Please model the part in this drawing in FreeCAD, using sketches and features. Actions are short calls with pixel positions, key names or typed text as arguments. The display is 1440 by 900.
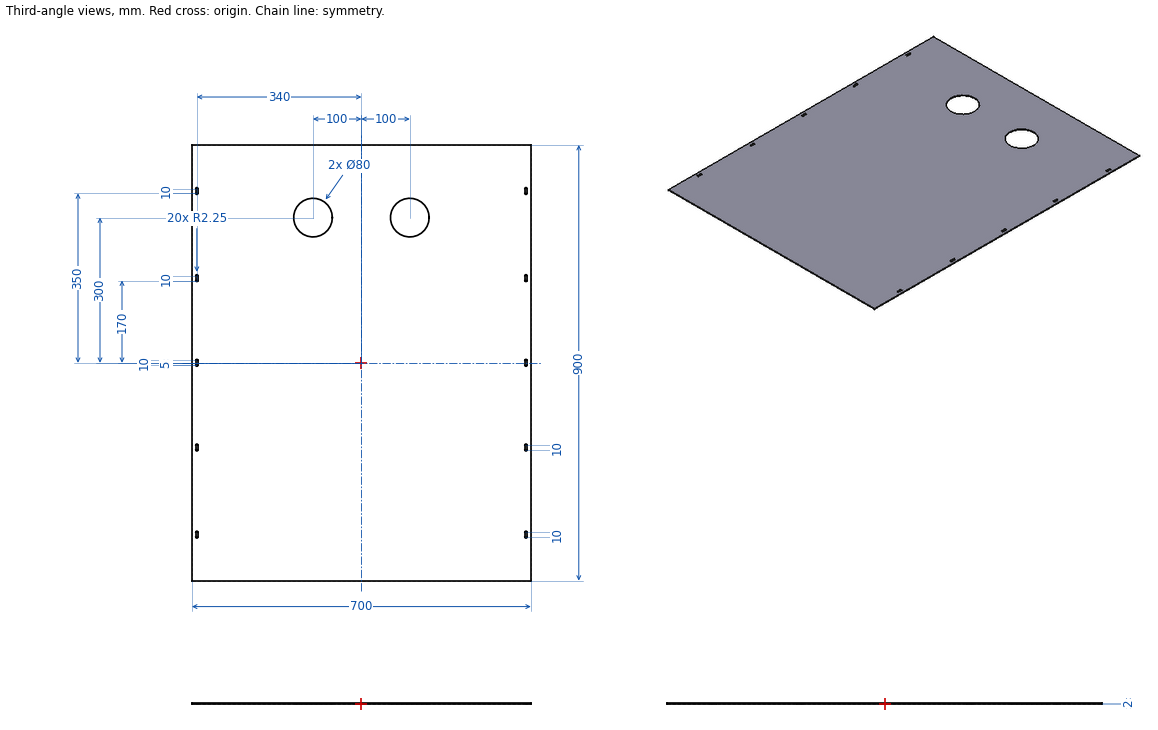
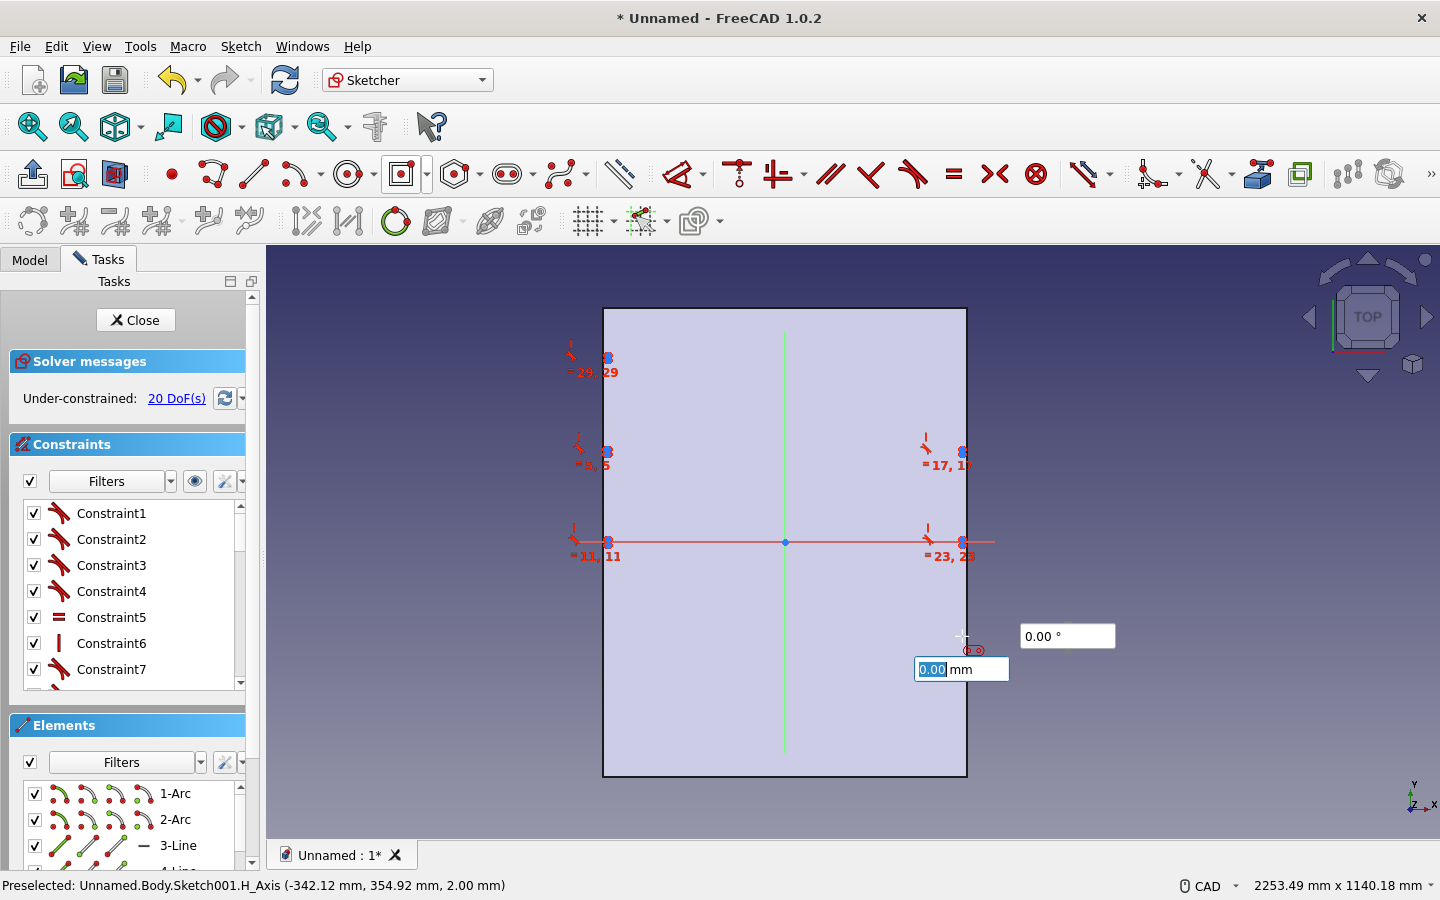
scroll(962, 631, up, 6)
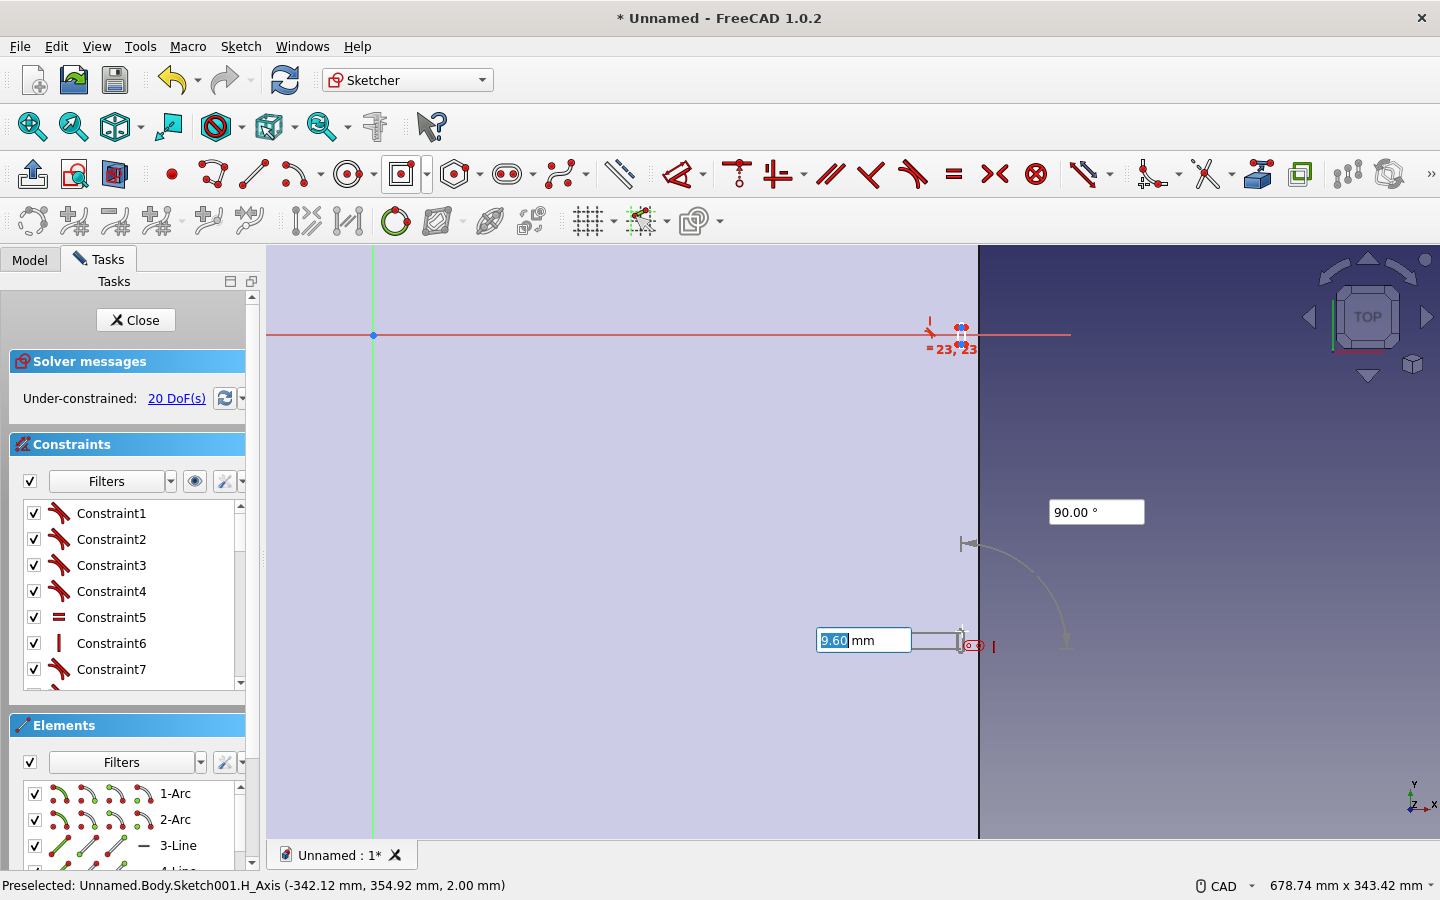
click(961, 630)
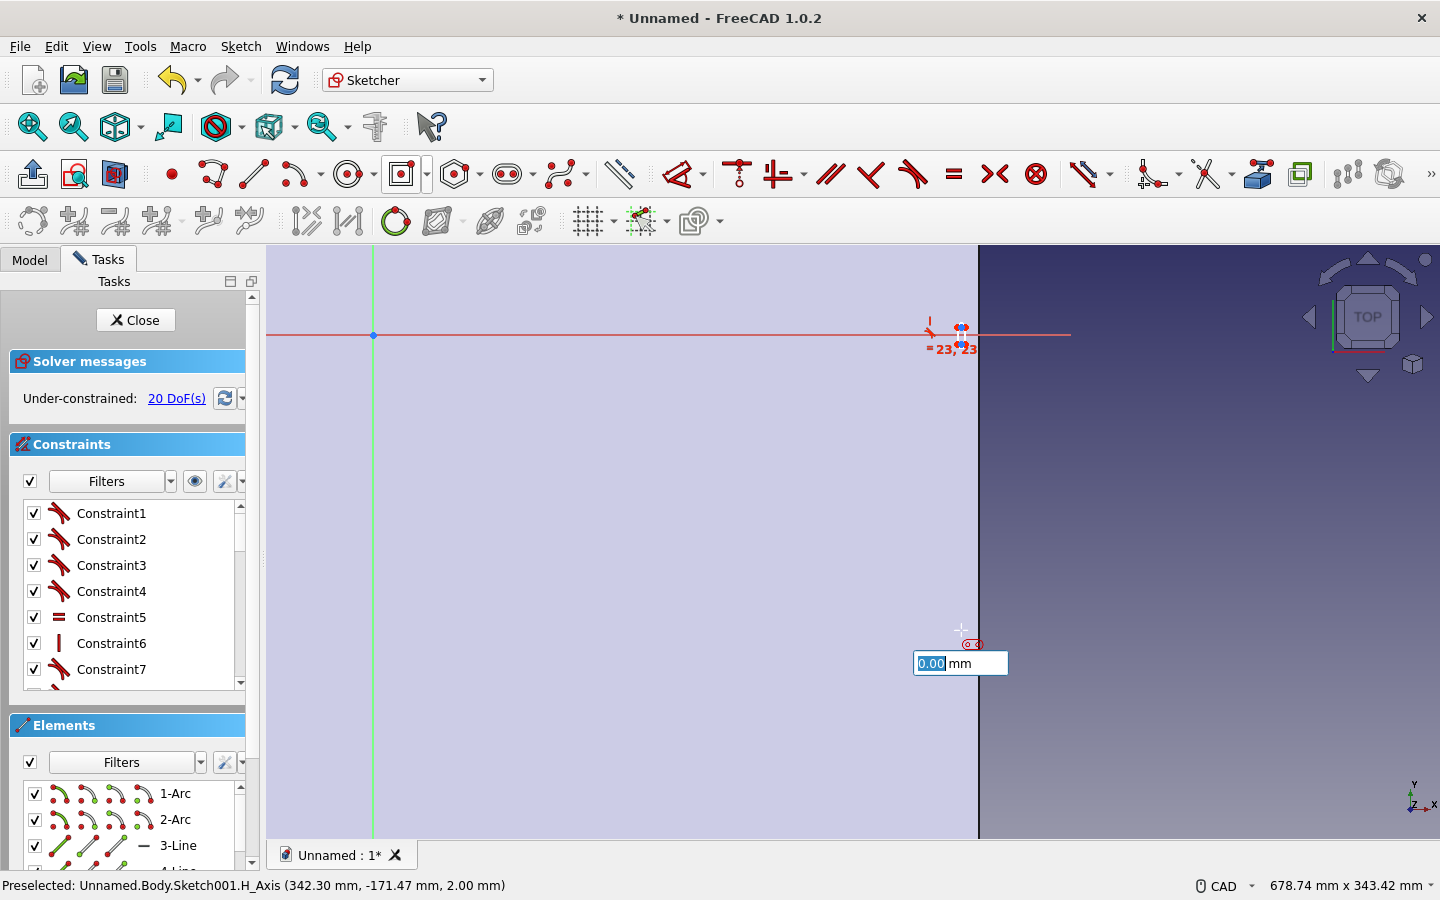
scroll(958, 638, up, 8)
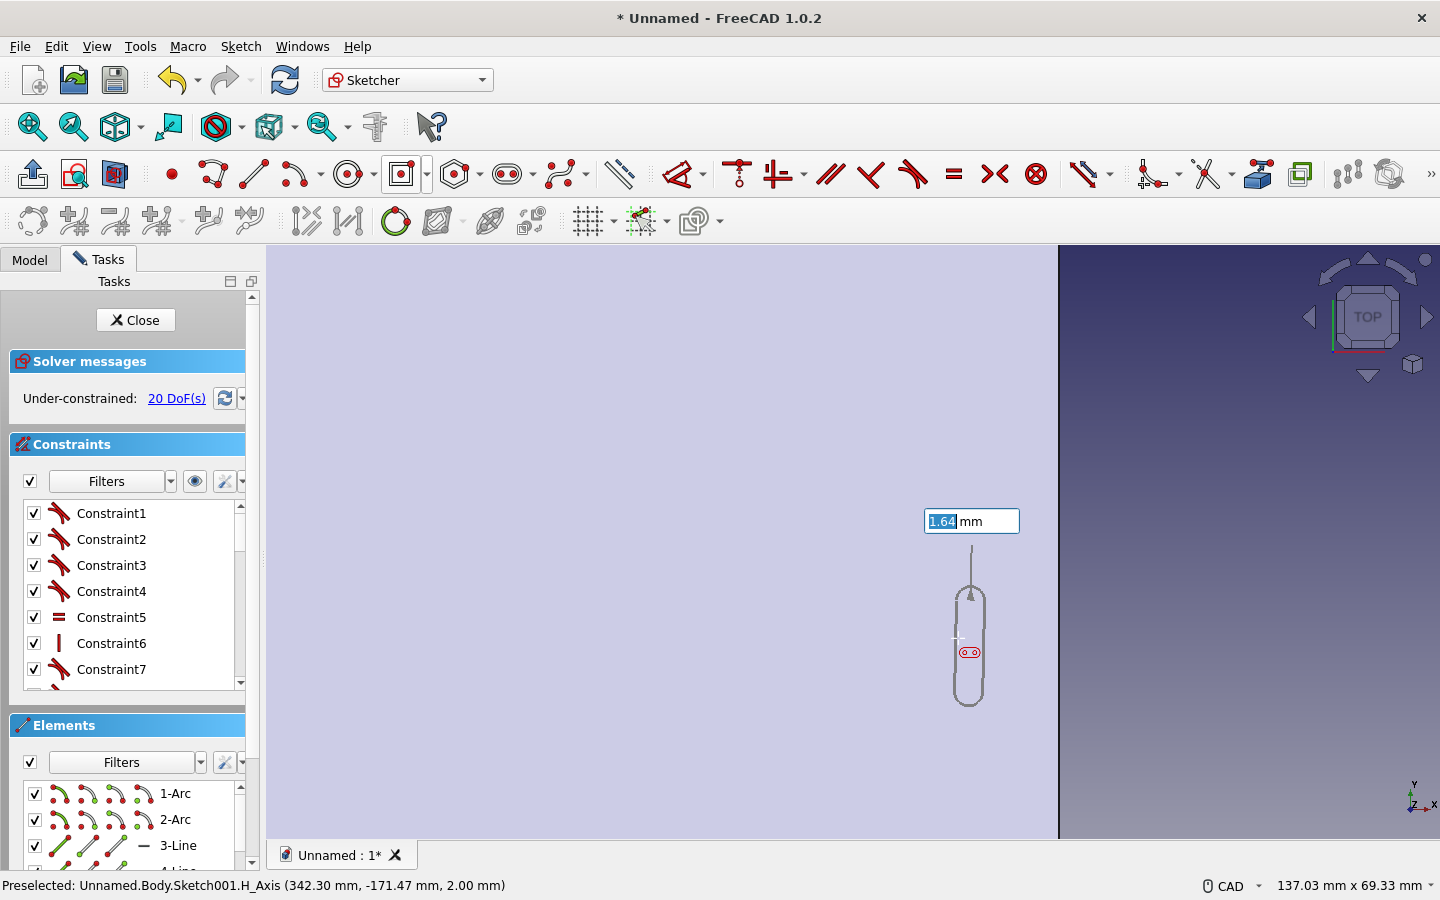
click(954, 636)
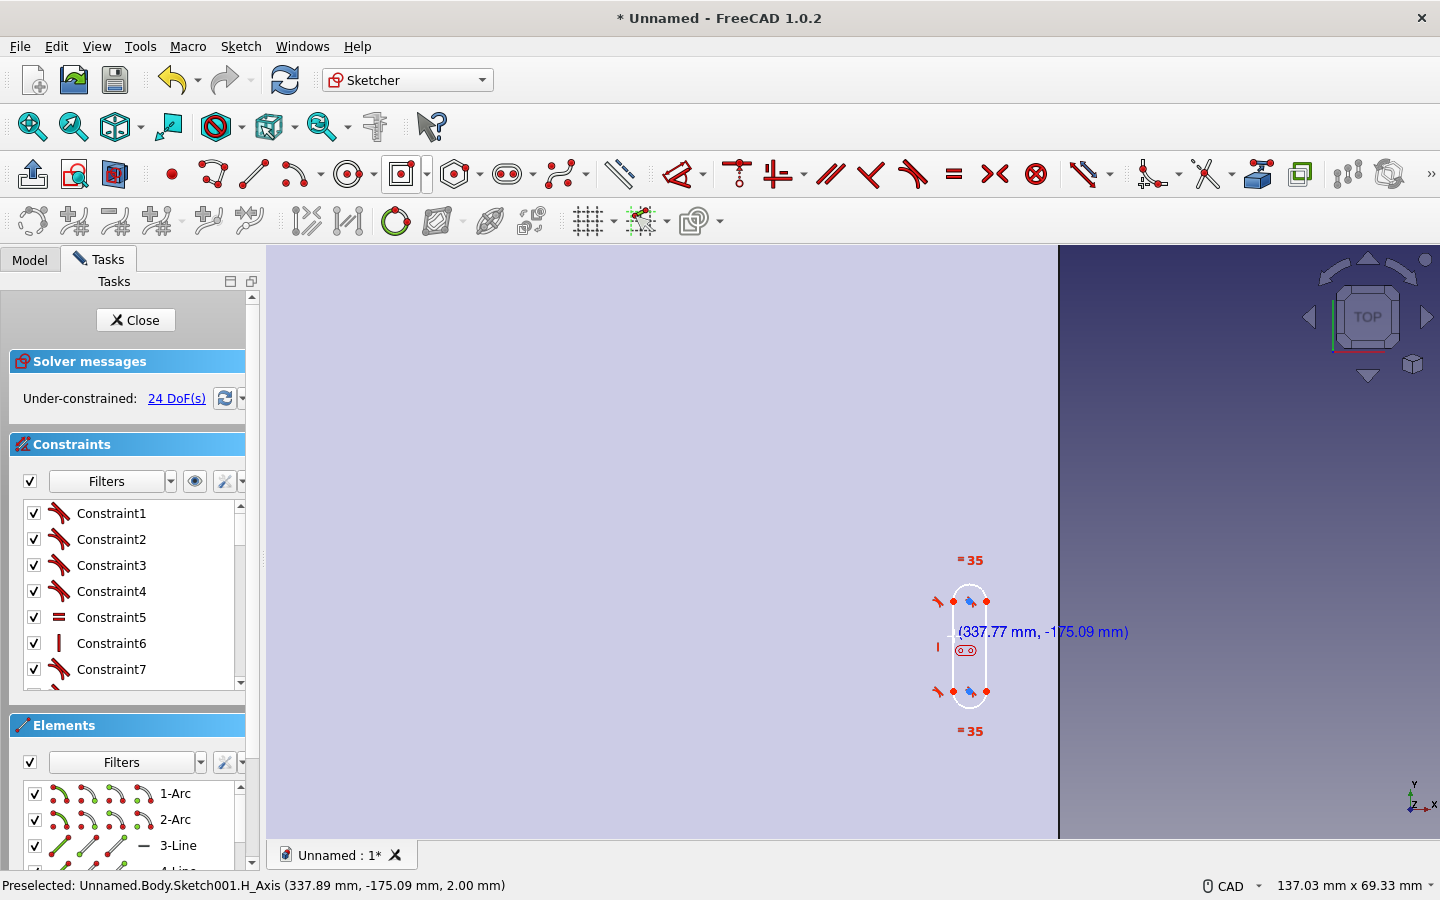
scroll(961, 633, down, 14)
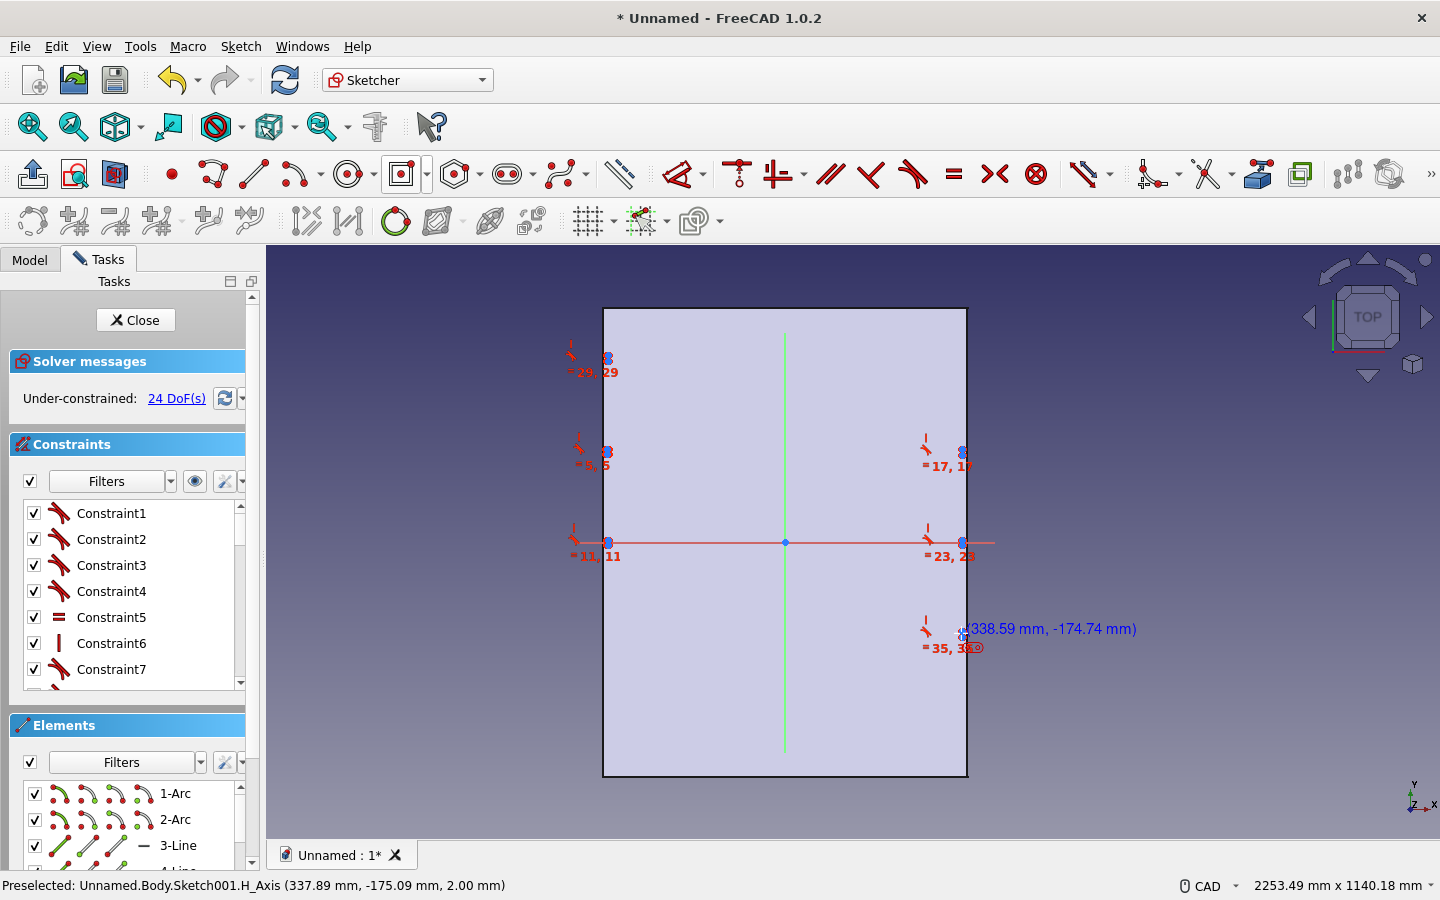
scroll(962, 360, up, 15)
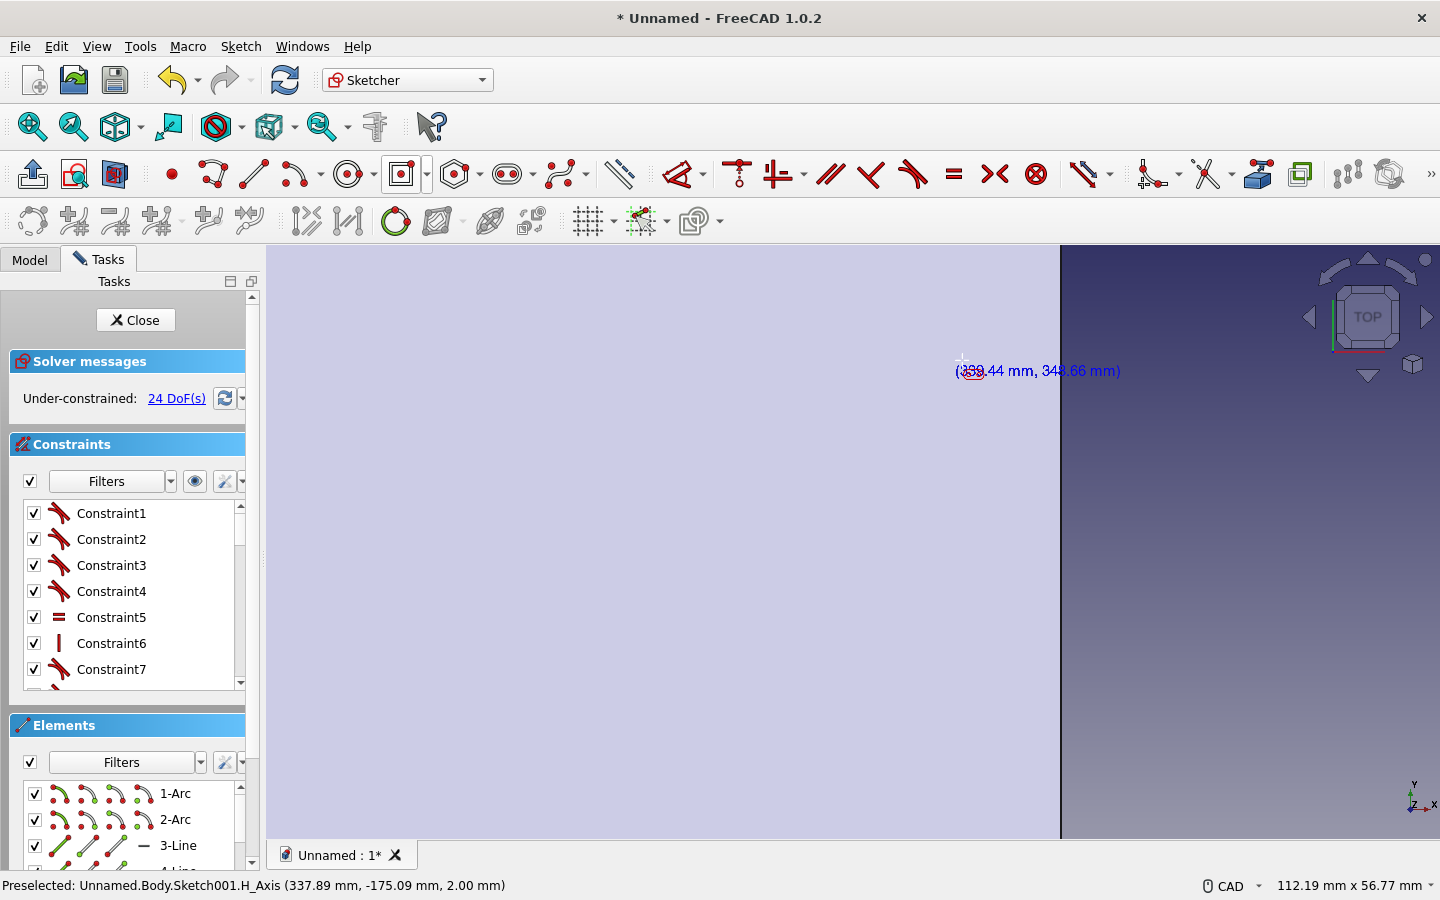
scroll(962, 360, down, 15)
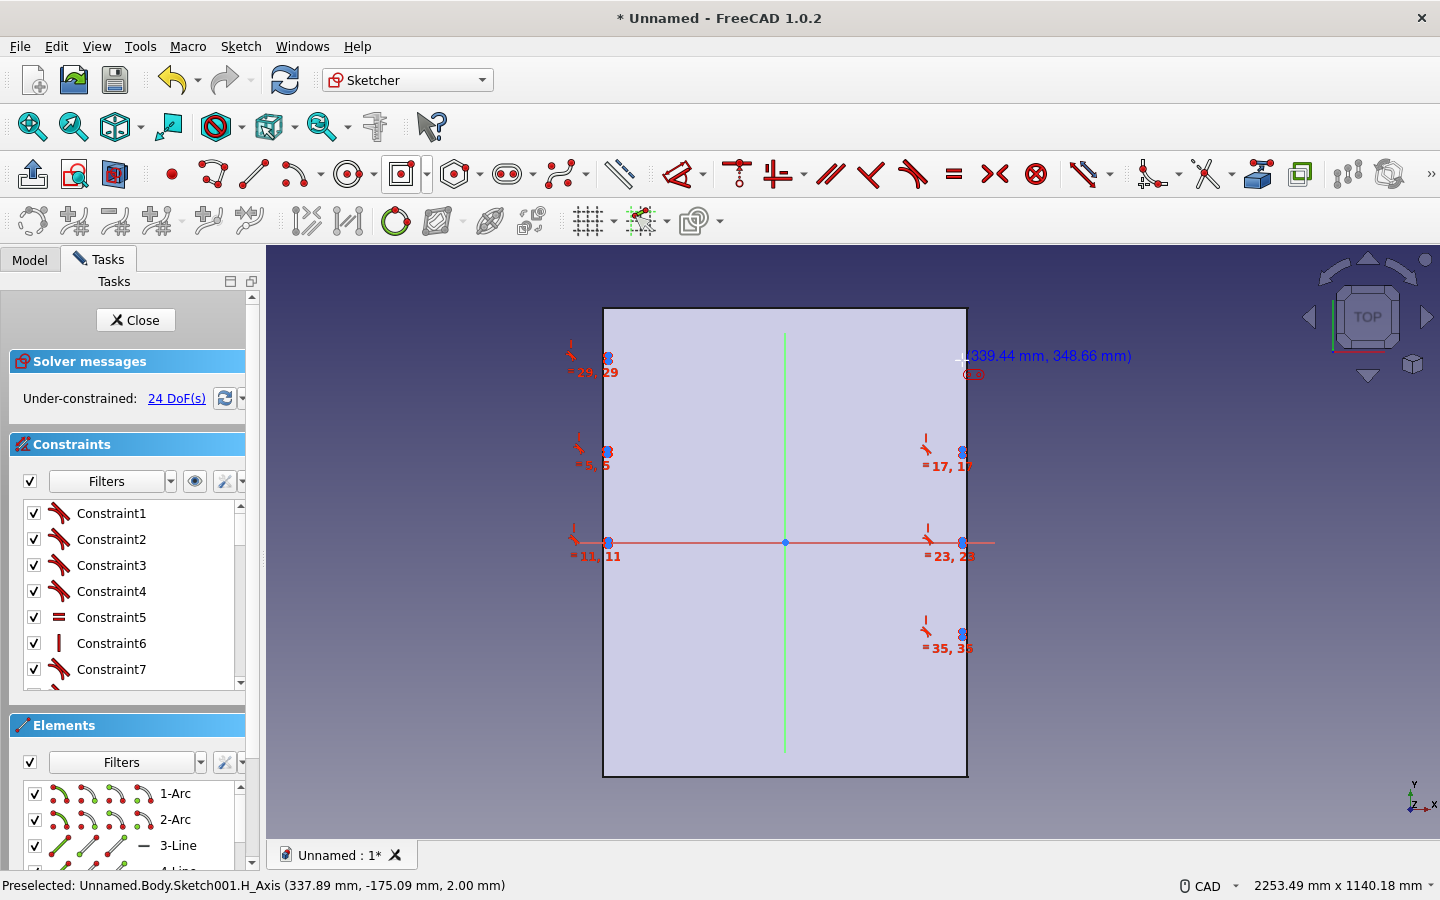
click(962, 360)